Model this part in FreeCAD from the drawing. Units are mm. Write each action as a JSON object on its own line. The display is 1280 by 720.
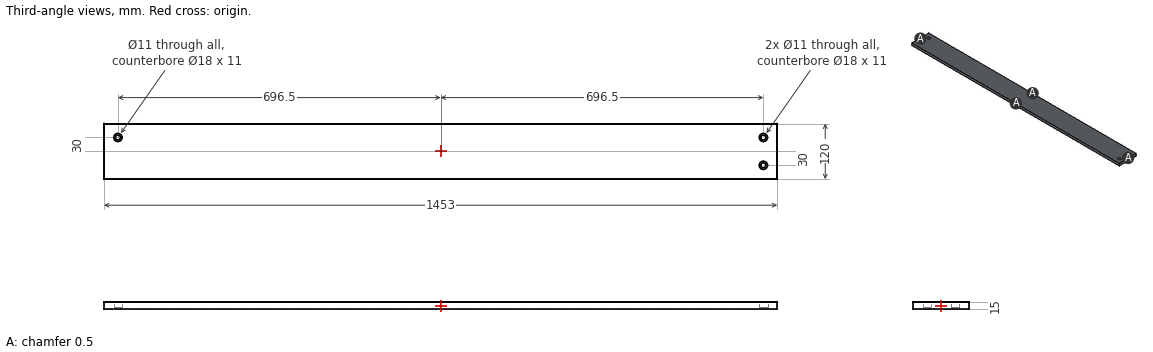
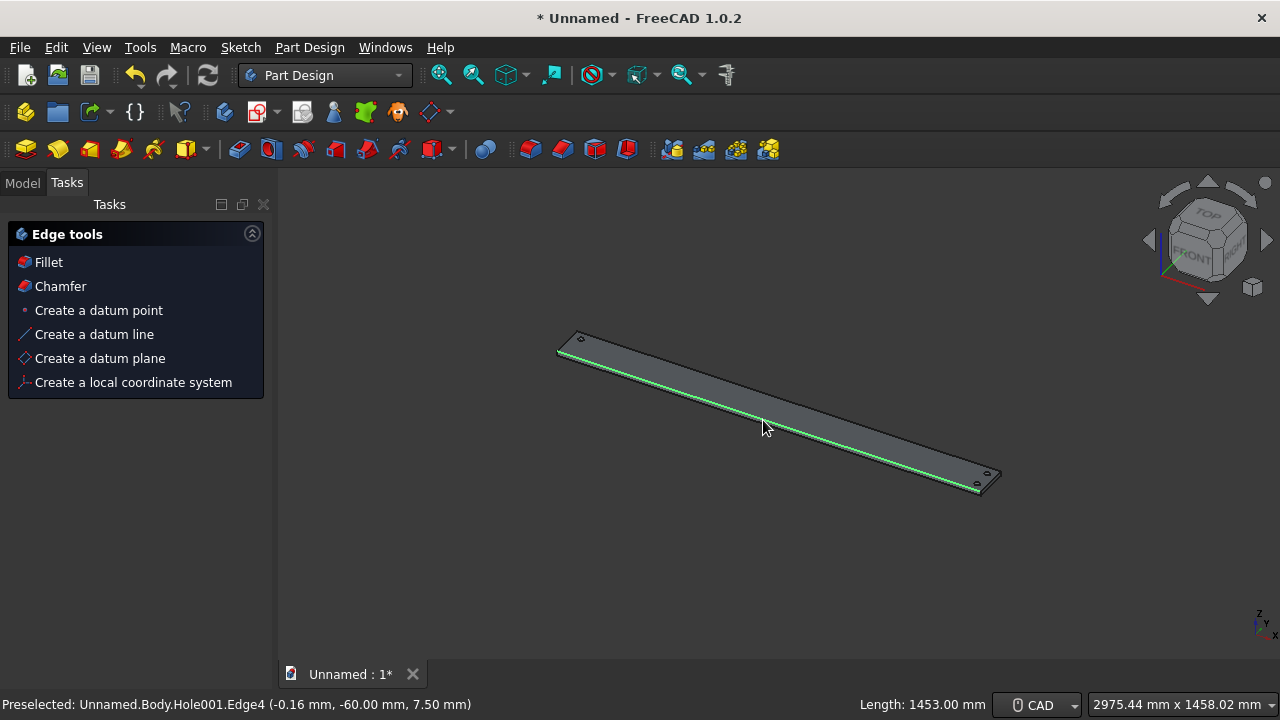
{"action": "left_click", "coordinate": [991, 481], "text": "ctrl"}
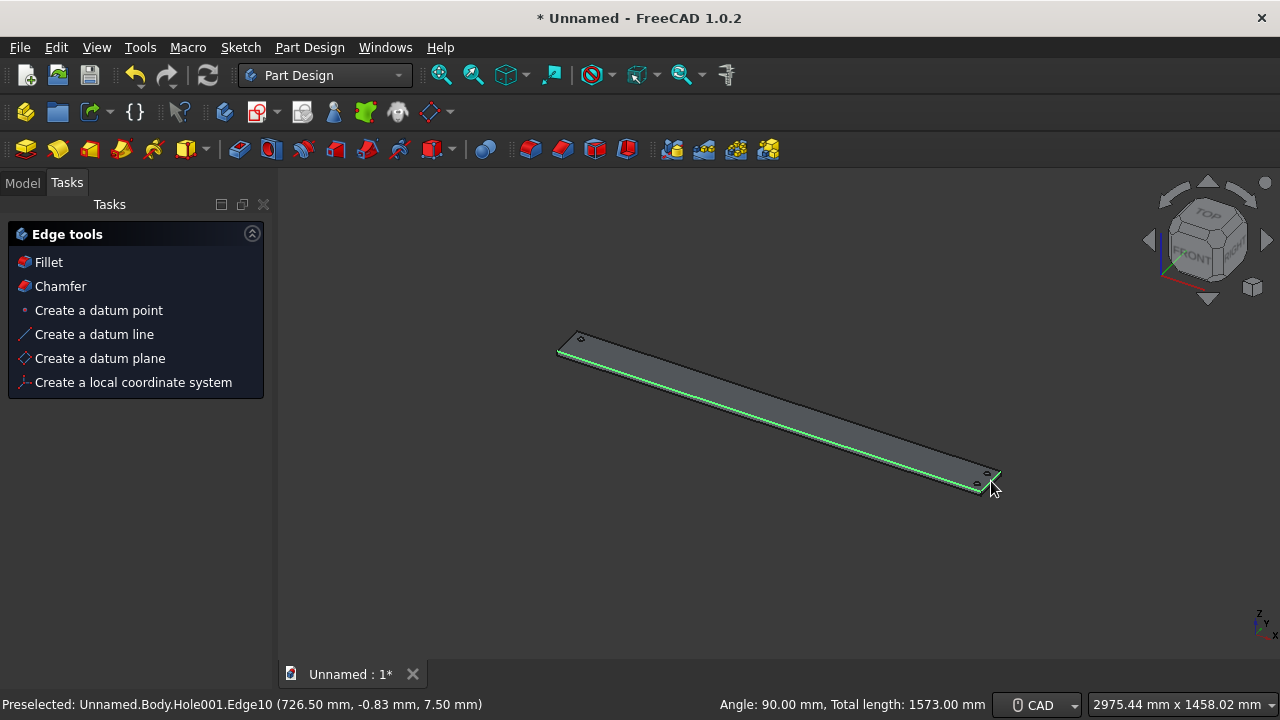
{"action": "key", "text": "0"}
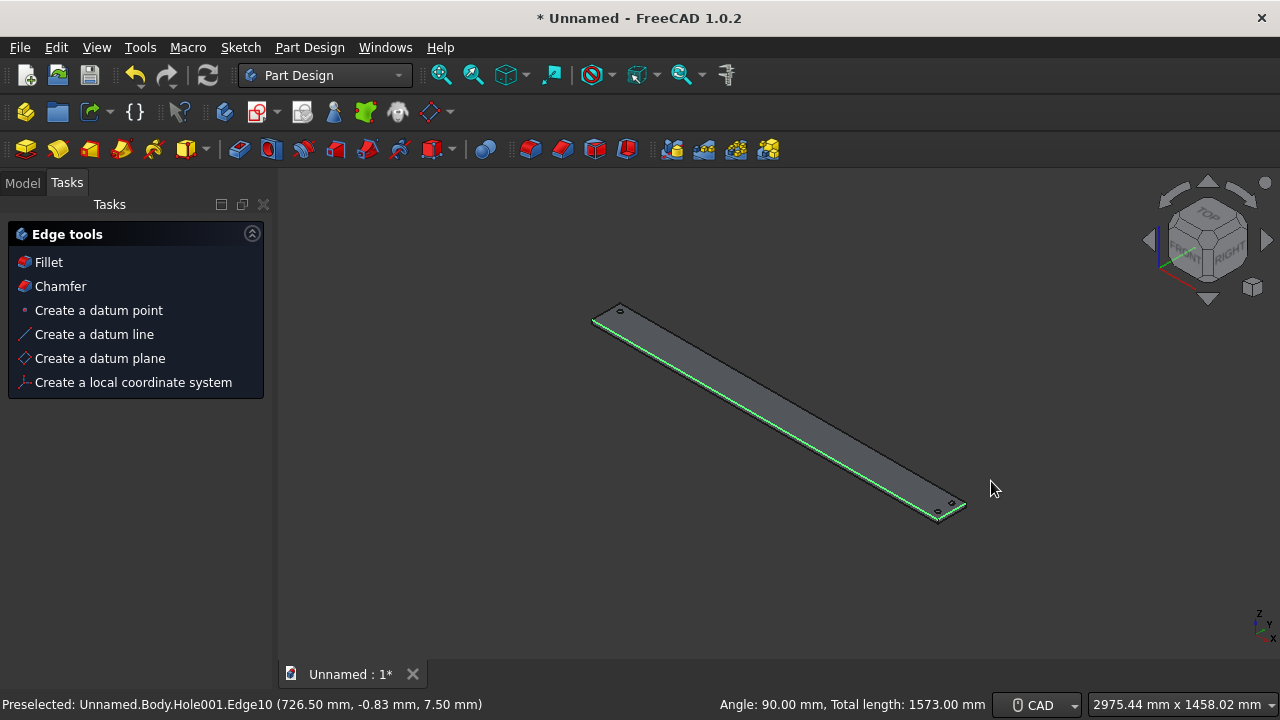
{"action": "key", "text": "2"}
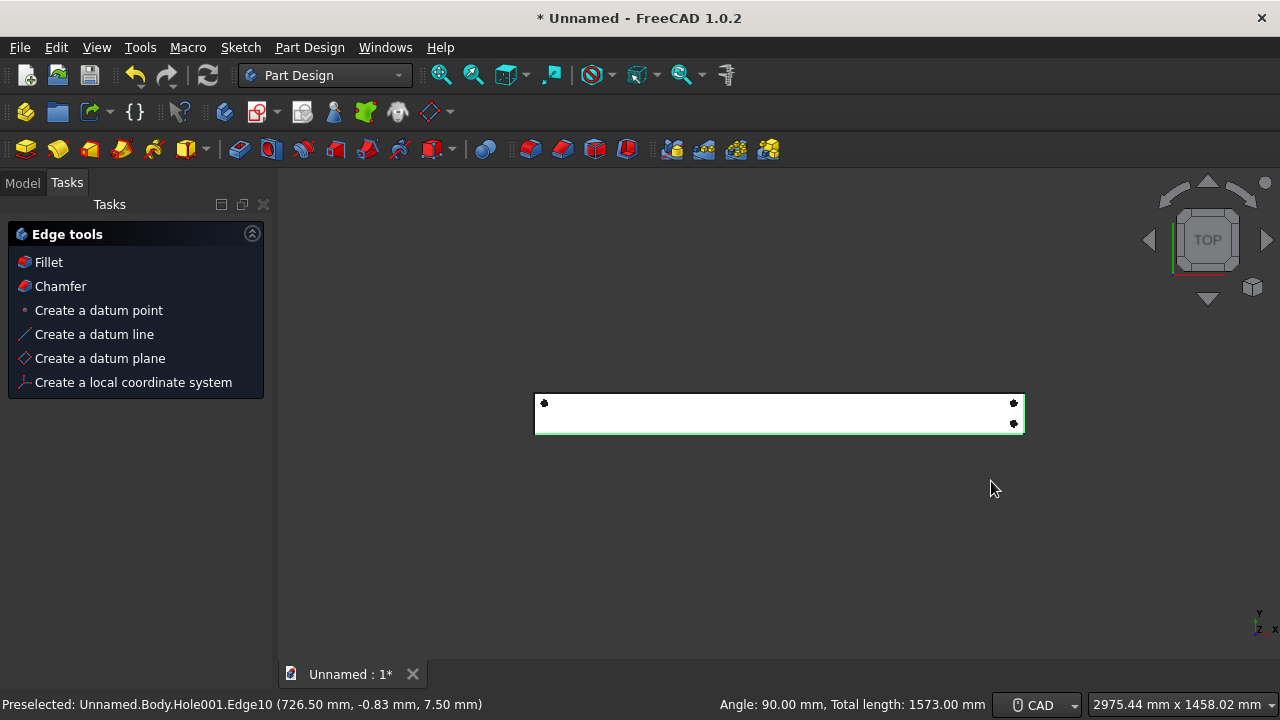
{"action": "left_click", "coordinate": [534, 413], "text": "ctrl"}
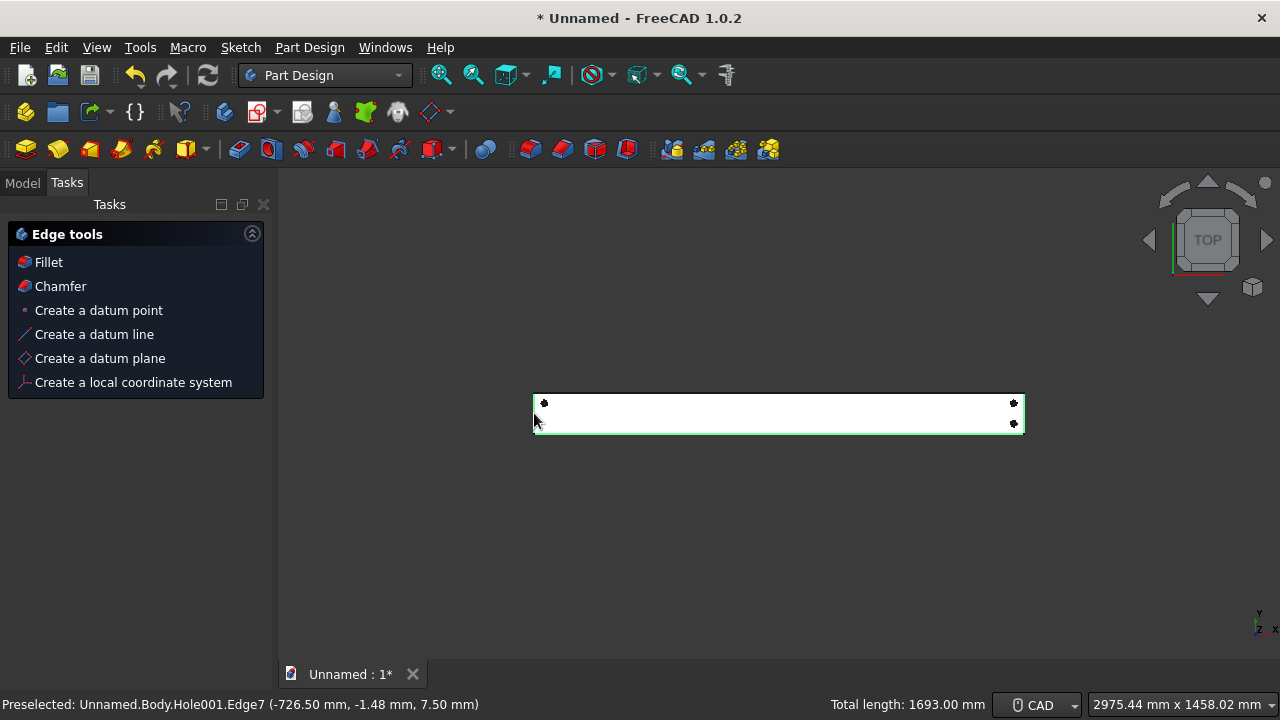
{"action": "left_click", "coordinate": [779, 392], "text": "ctrl"}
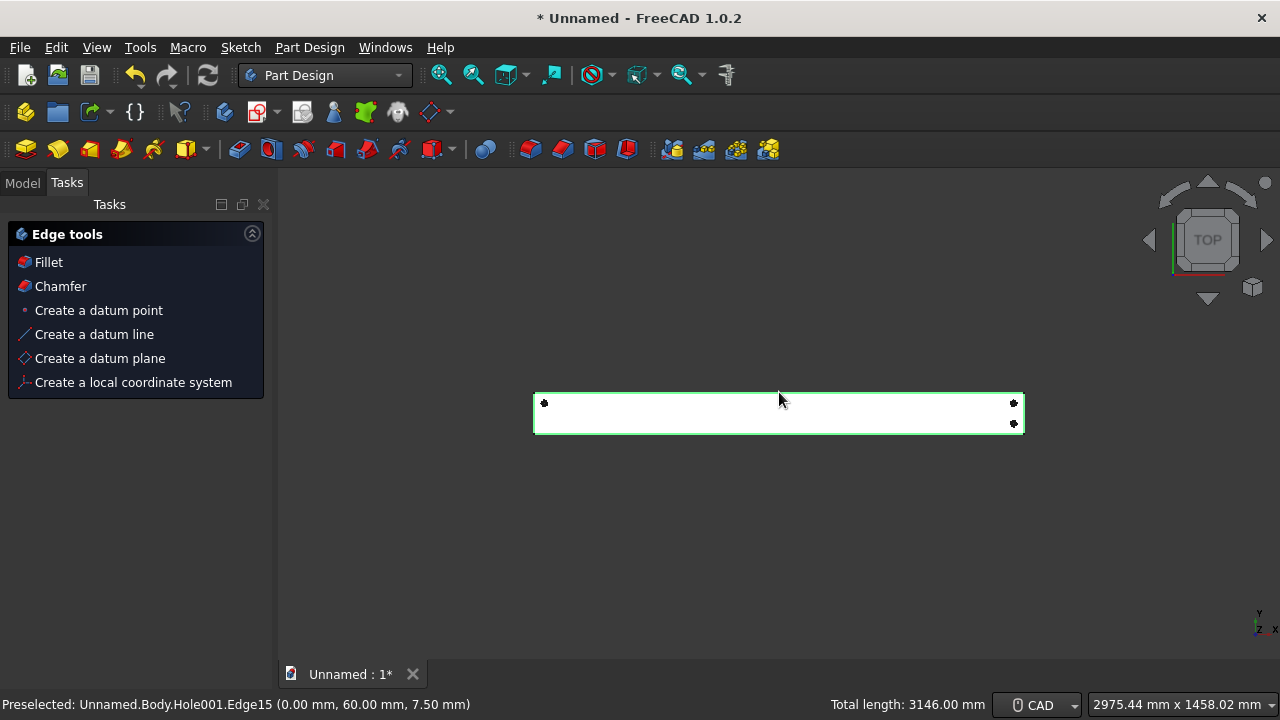
{"action": "left_click", "coordinate": [564, 150]}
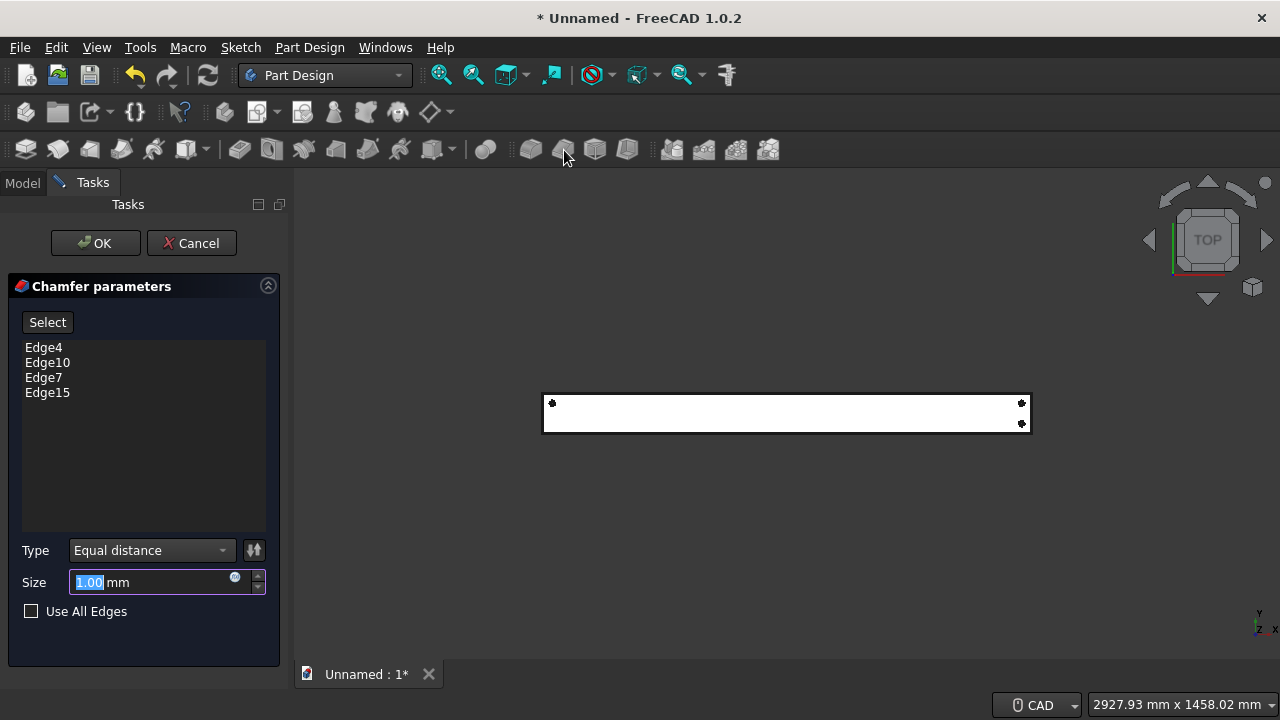
{"action": "type", "text": "0.5"}
{"action": "key", "text": "Tab"}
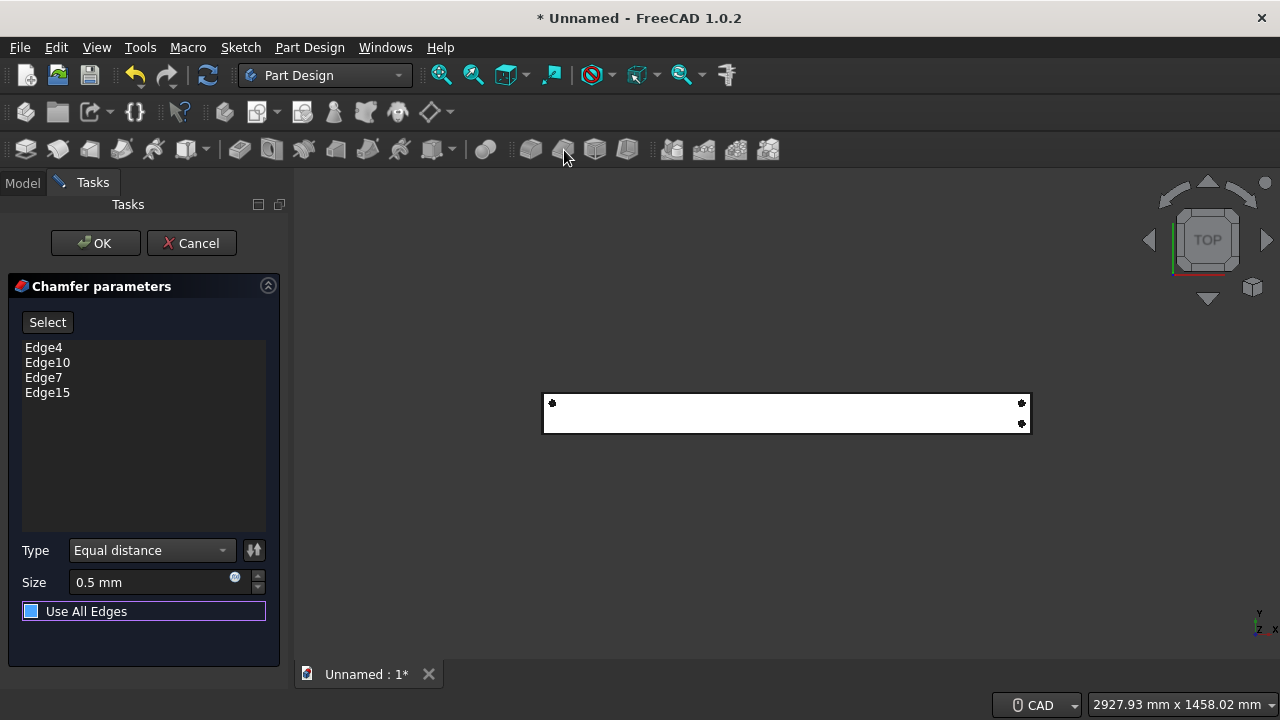
{"action": "left_click", "coordinate": [96, 243]}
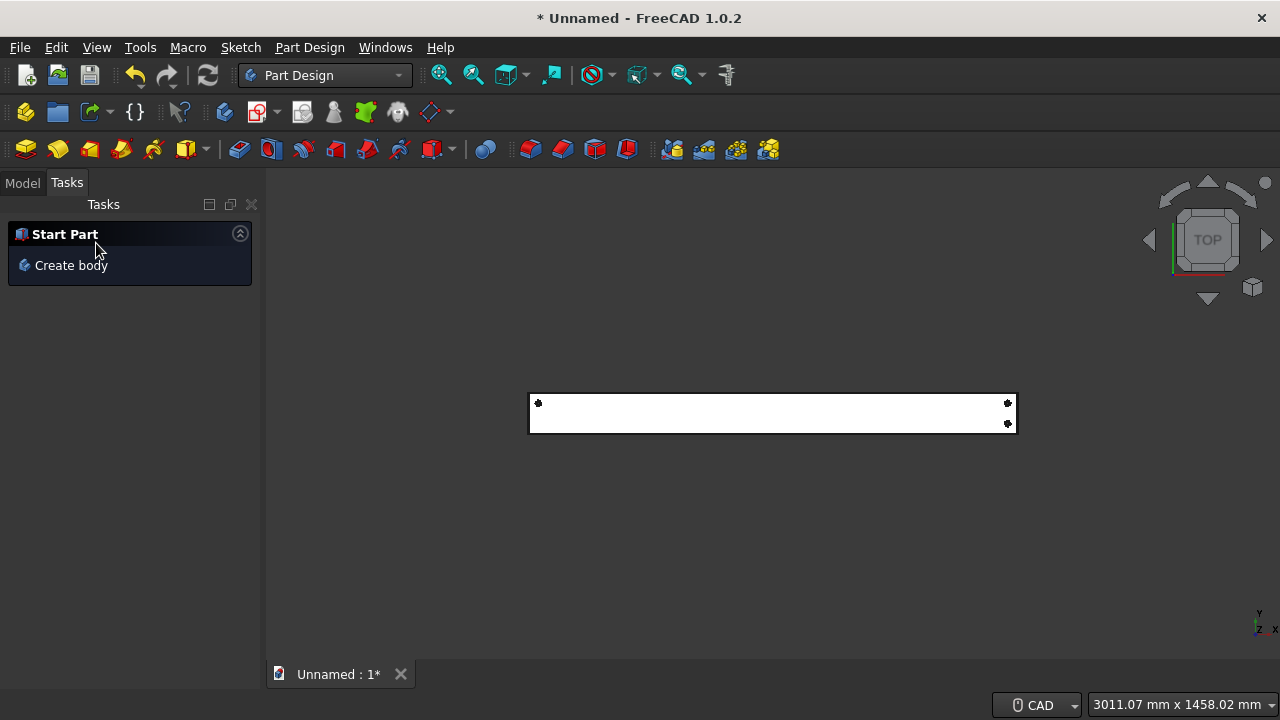
{"action": "key", "text": "0"}